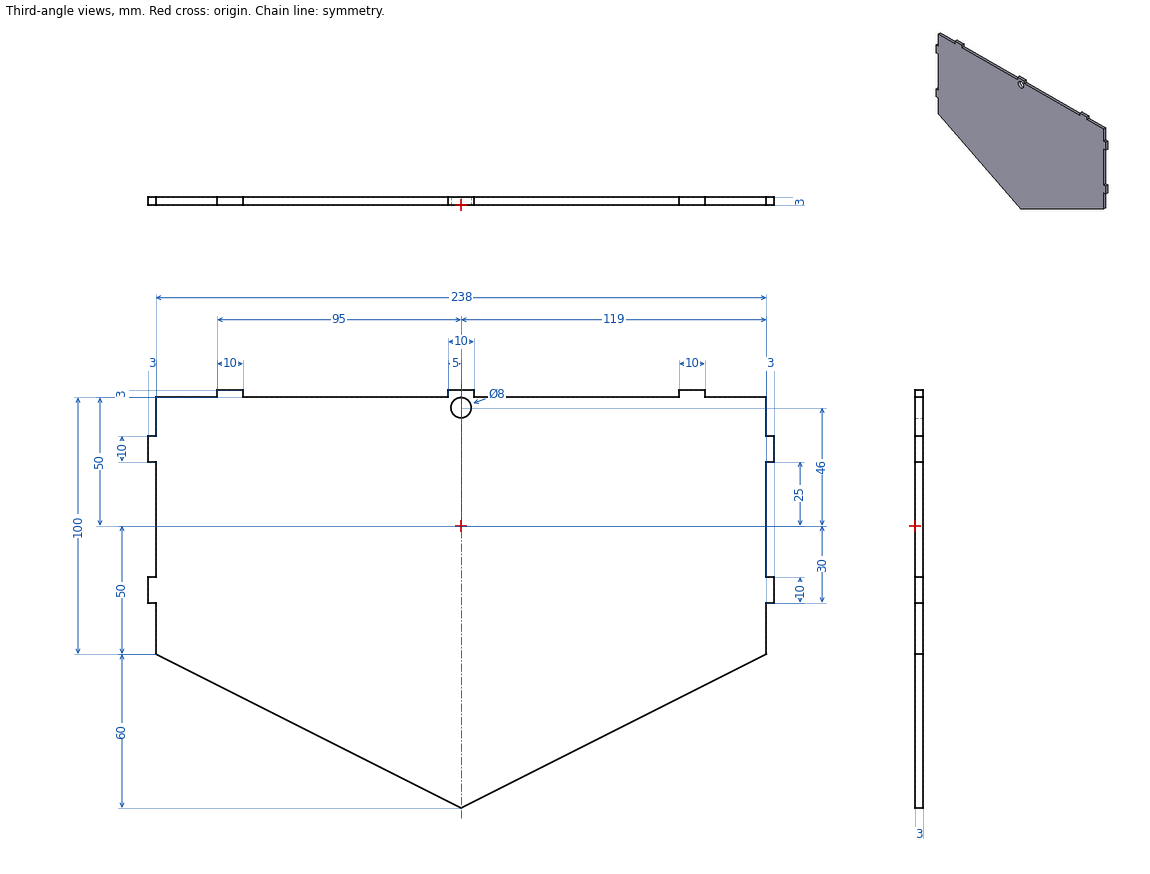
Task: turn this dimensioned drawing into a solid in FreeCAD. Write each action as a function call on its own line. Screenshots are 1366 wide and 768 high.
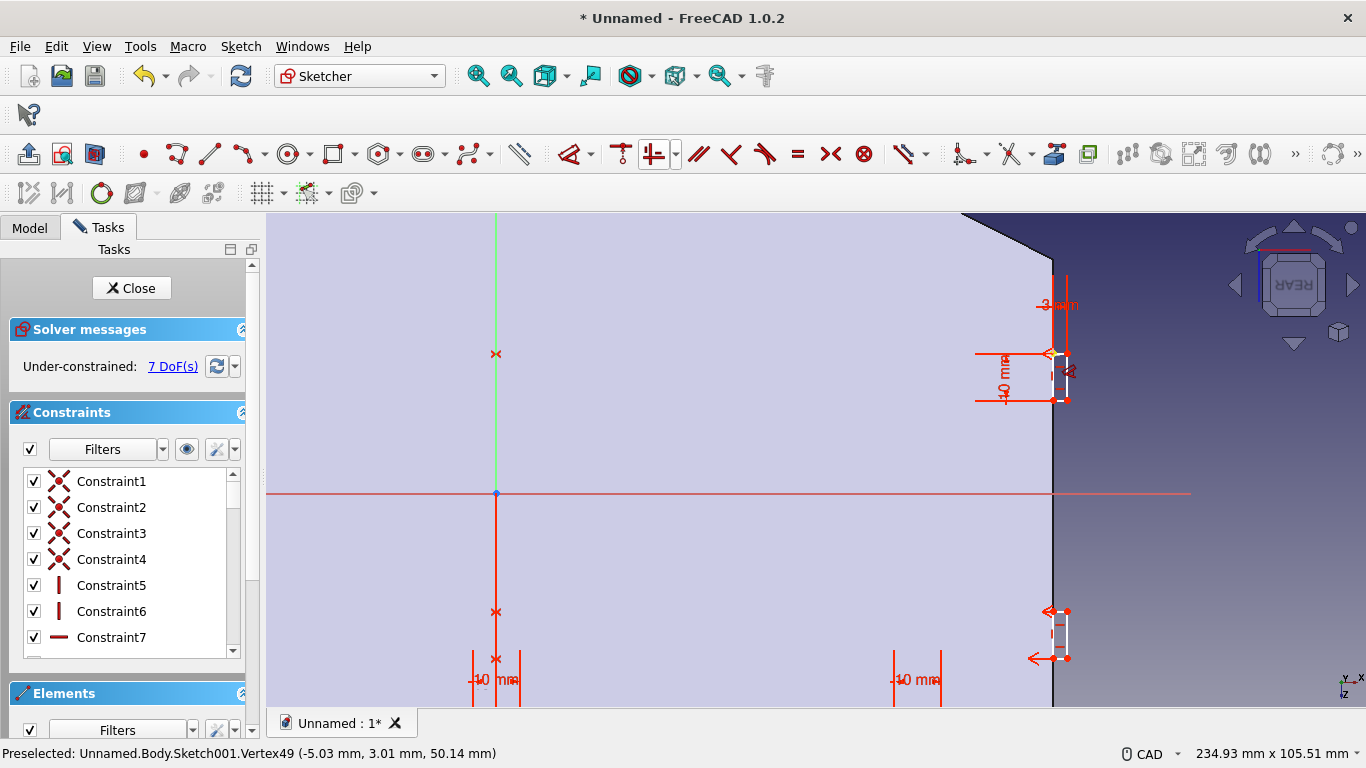
click(1053, 354)
click(1087, 424)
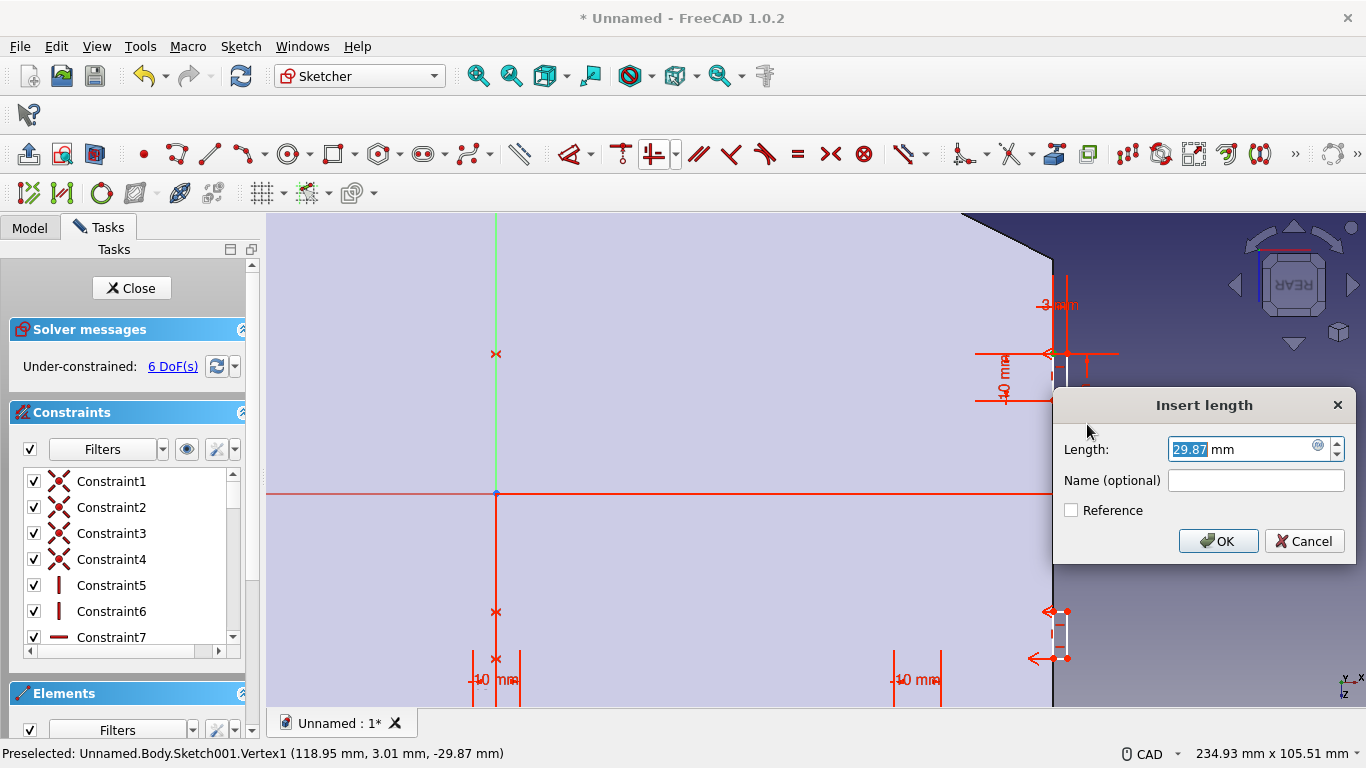
text(30)
key(Return)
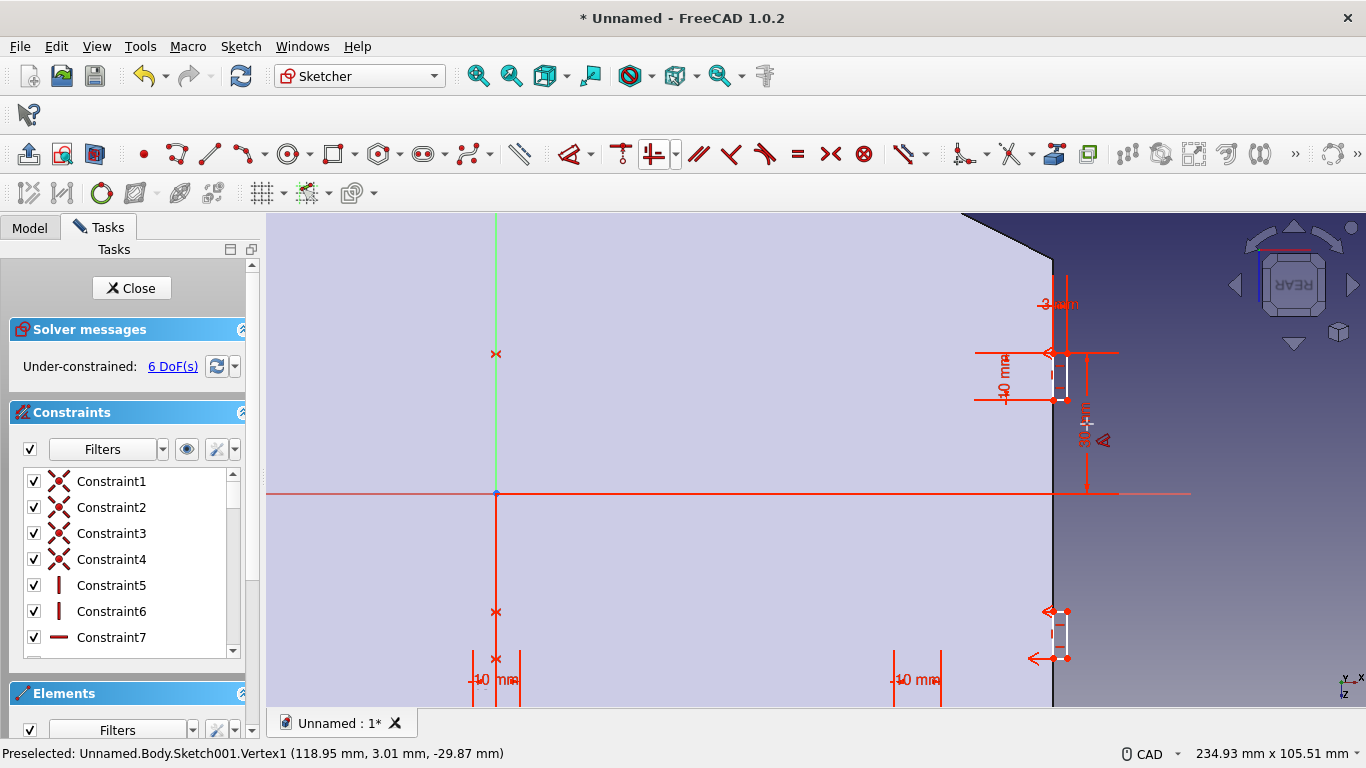
click(1053, 612)
click(1087, 553)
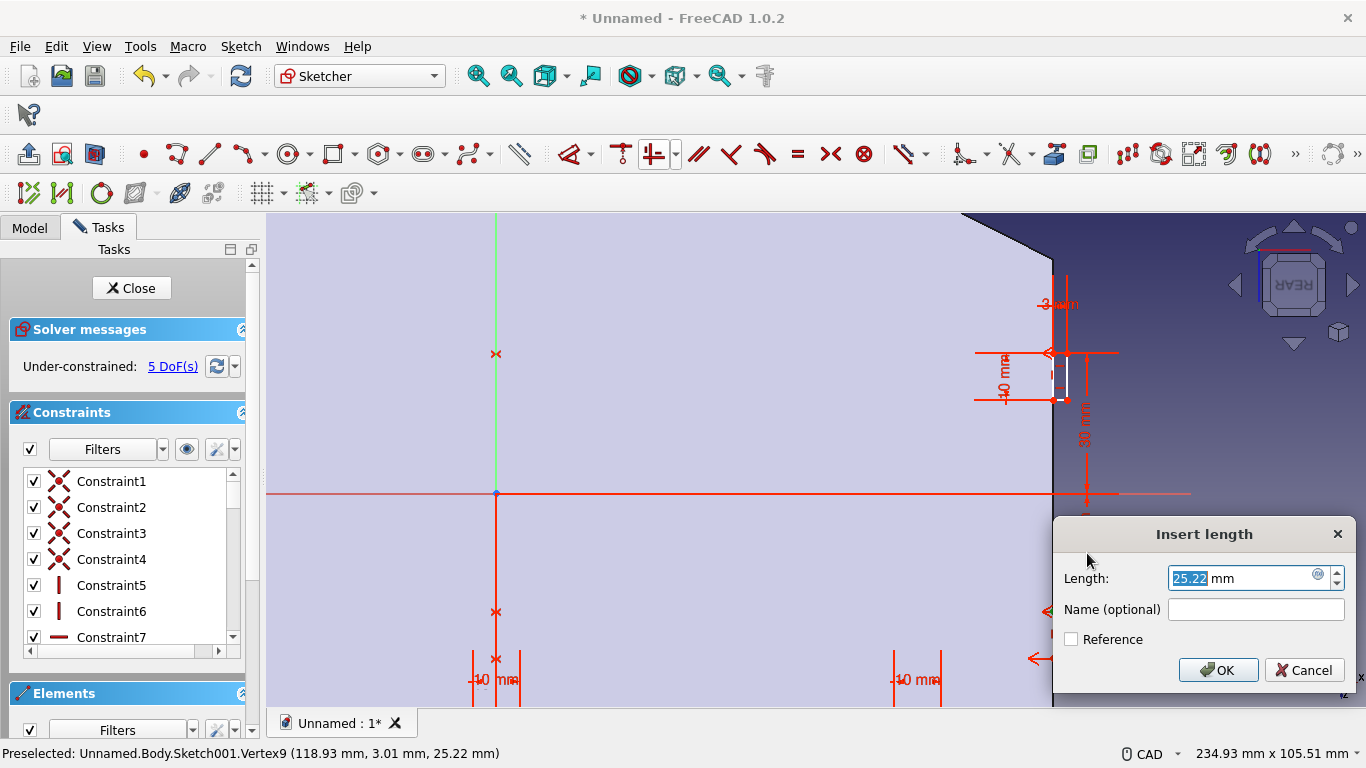
text(25)
key(Return)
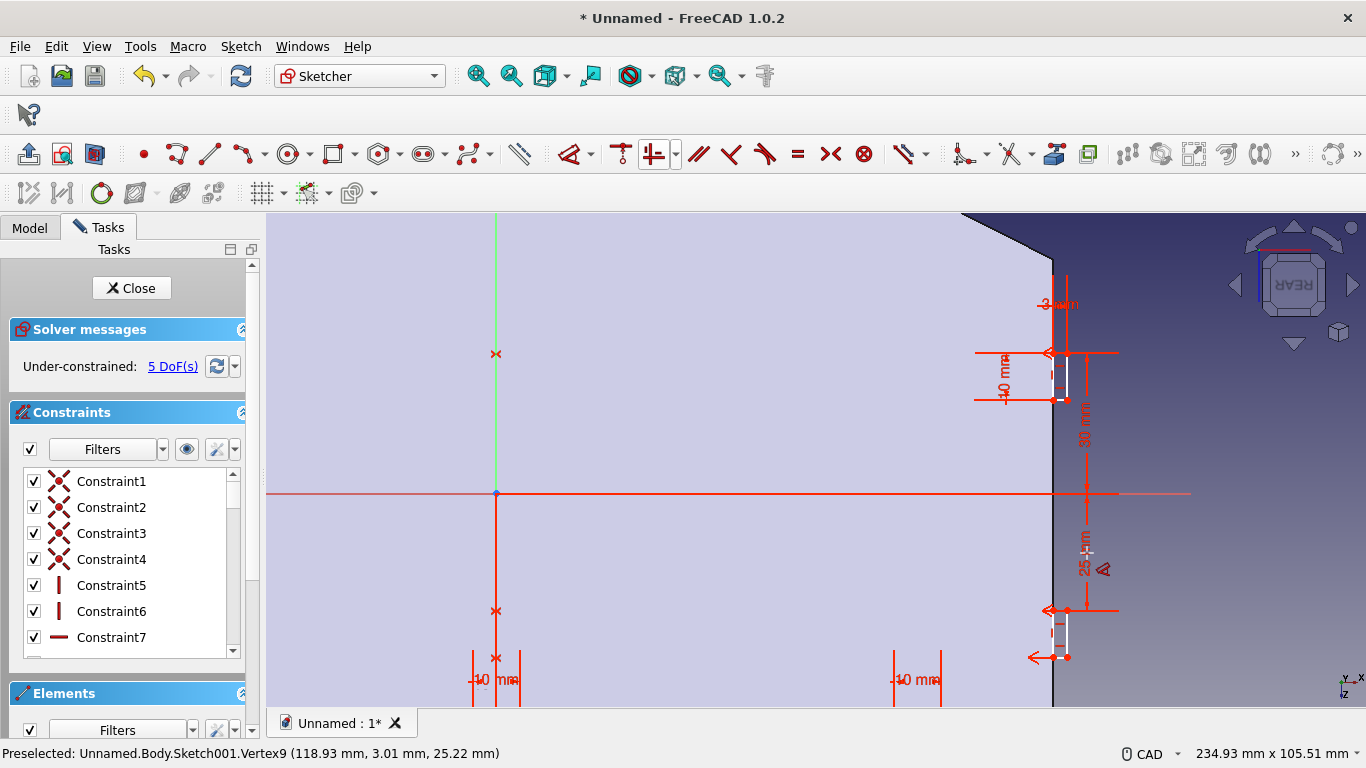
scroll(1053, 354, down, 3)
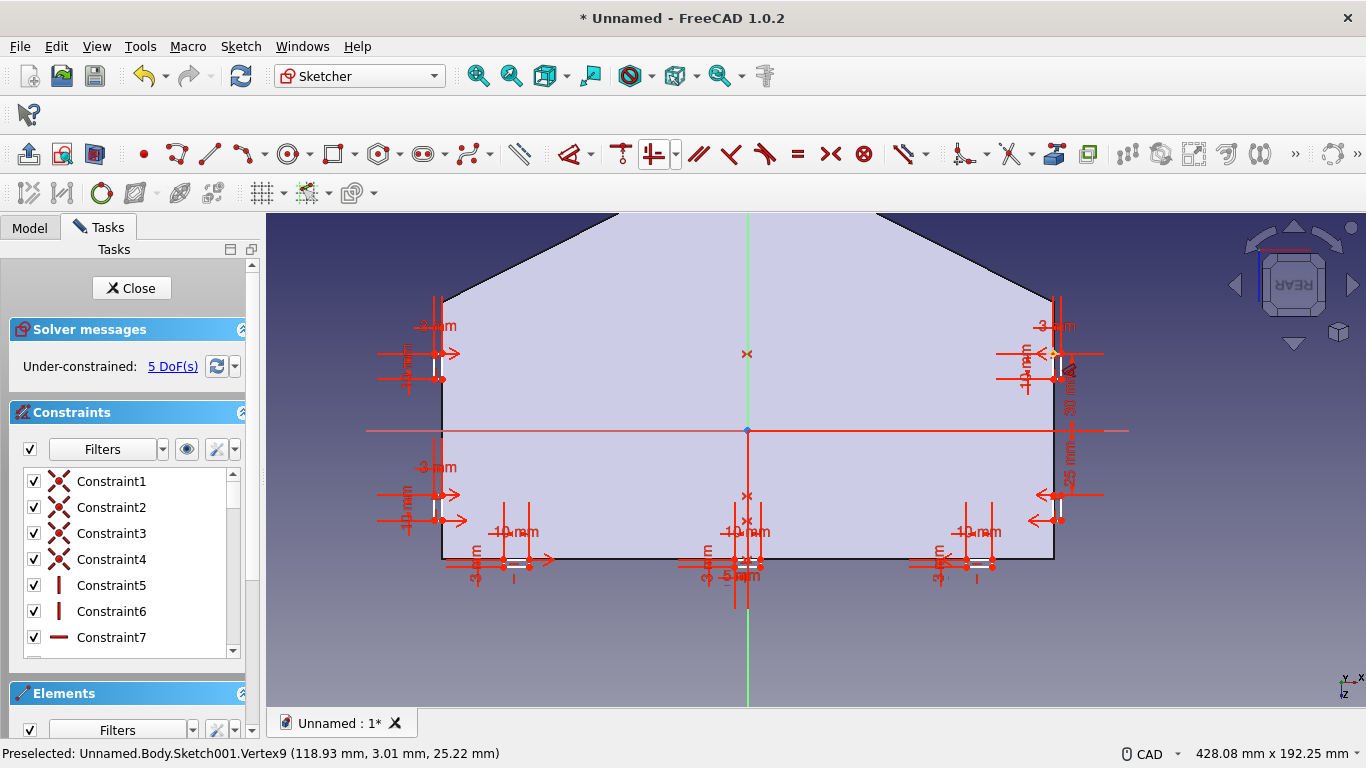
scroll(504, 560, up, 3)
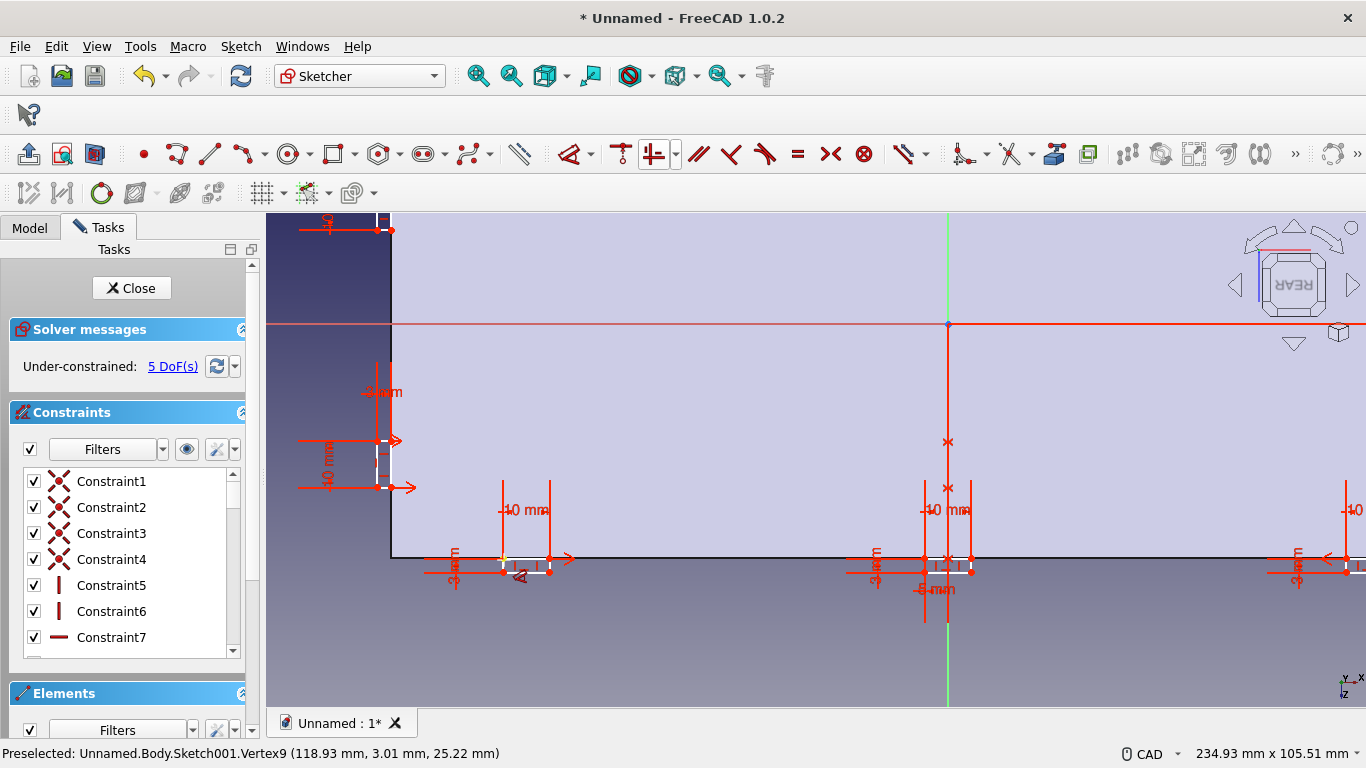
click(503, 559)
click(726, 593)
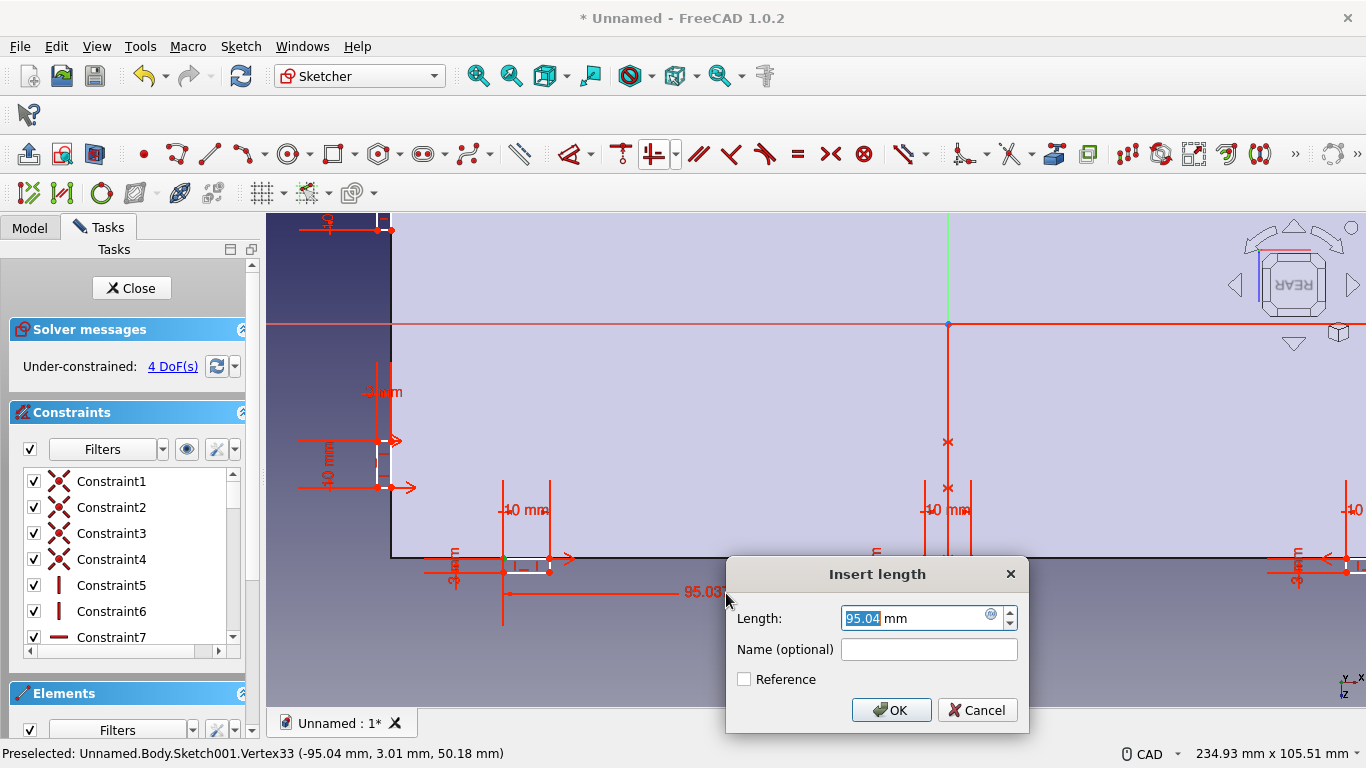
text(95)
key(Return)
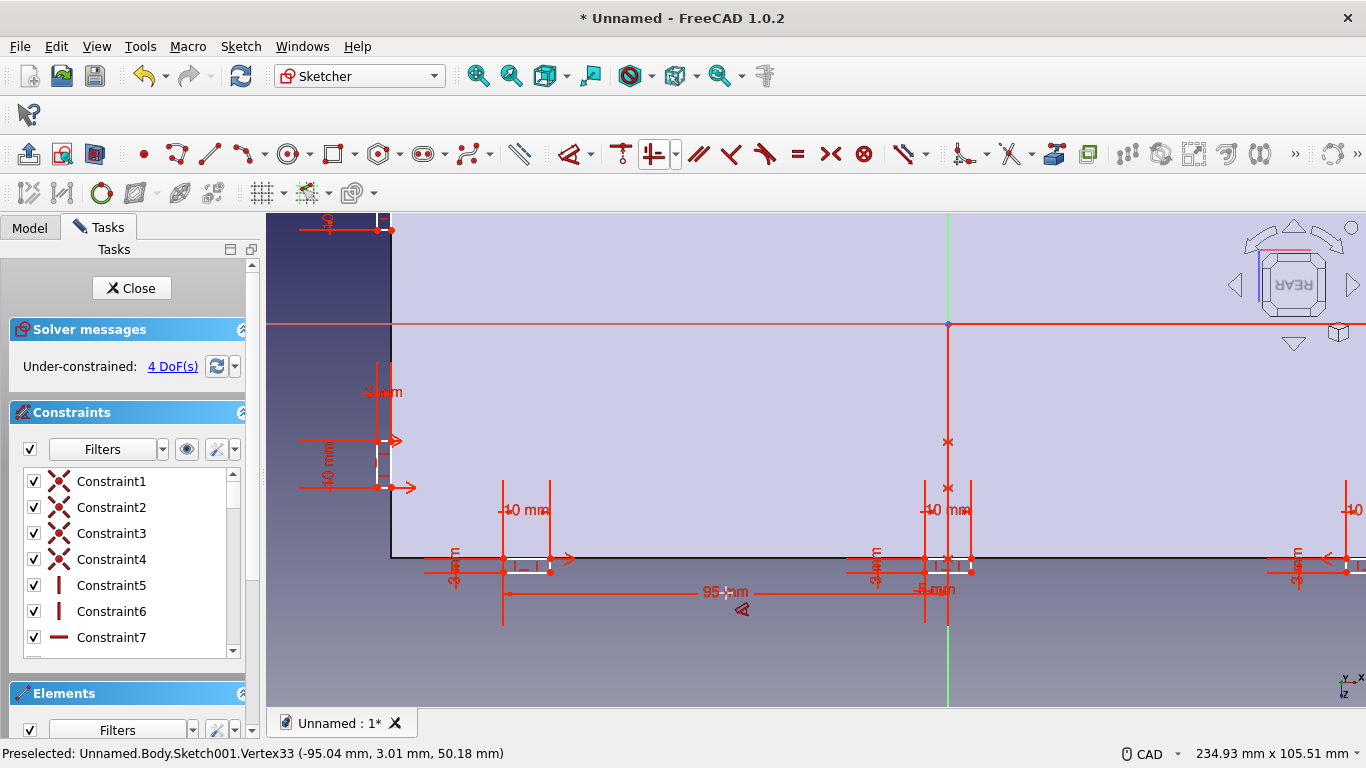
click(503, 559)
click(469, 441)